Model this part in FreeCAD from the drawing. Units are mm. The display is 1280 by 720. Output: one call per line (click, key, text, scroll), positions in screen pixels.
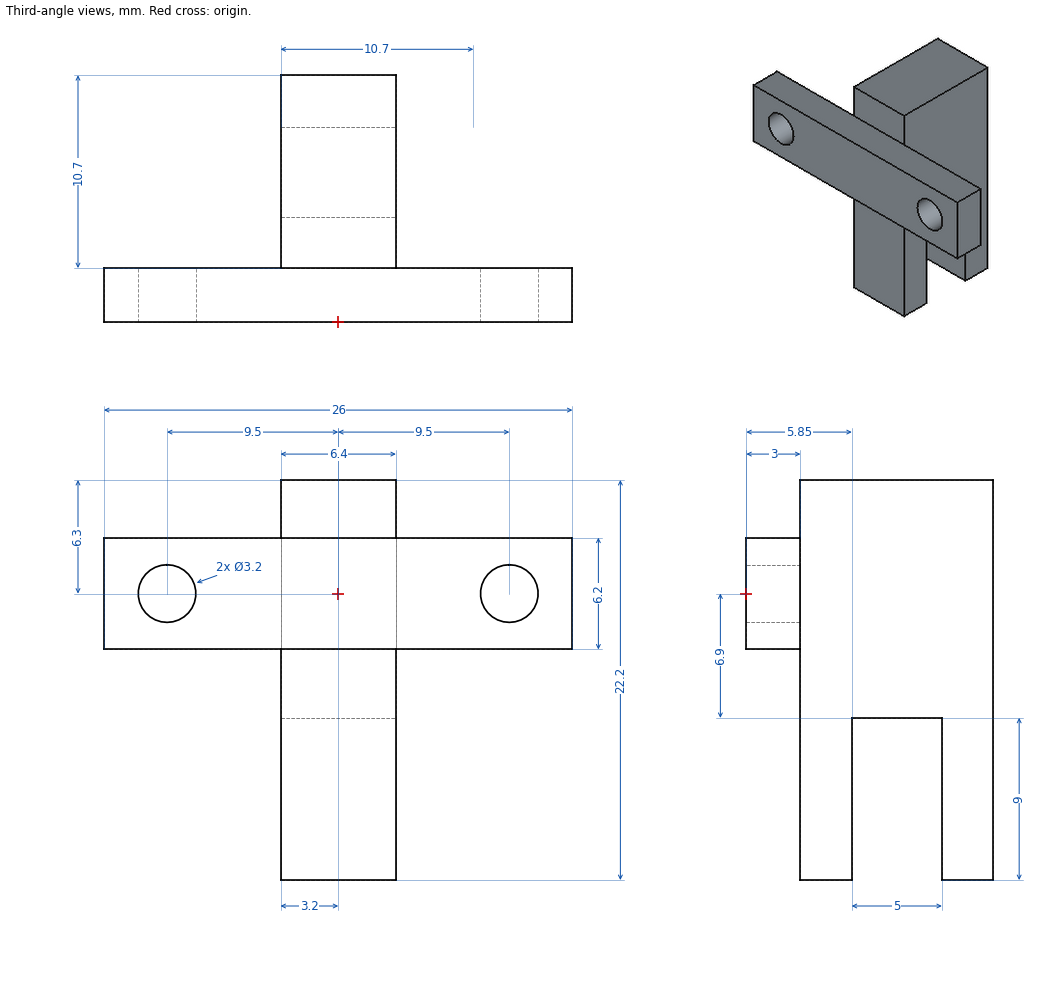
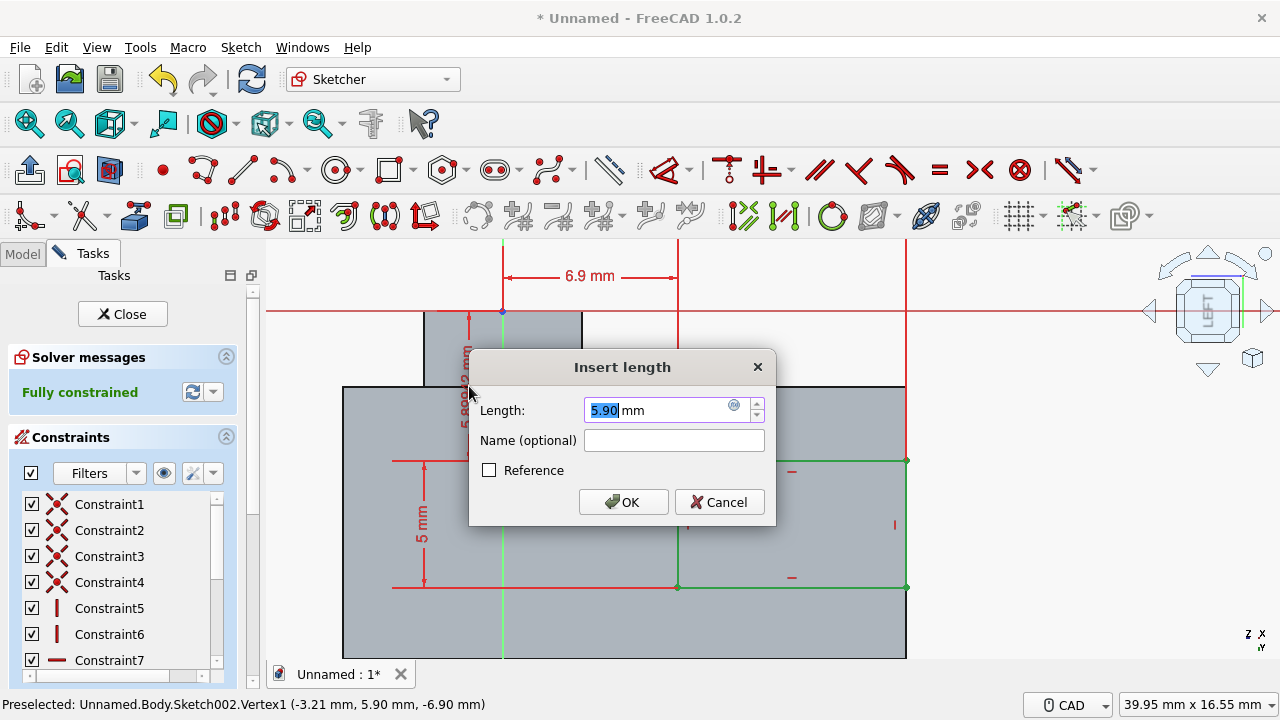
text(5.85)
key(Return)
key(Escape)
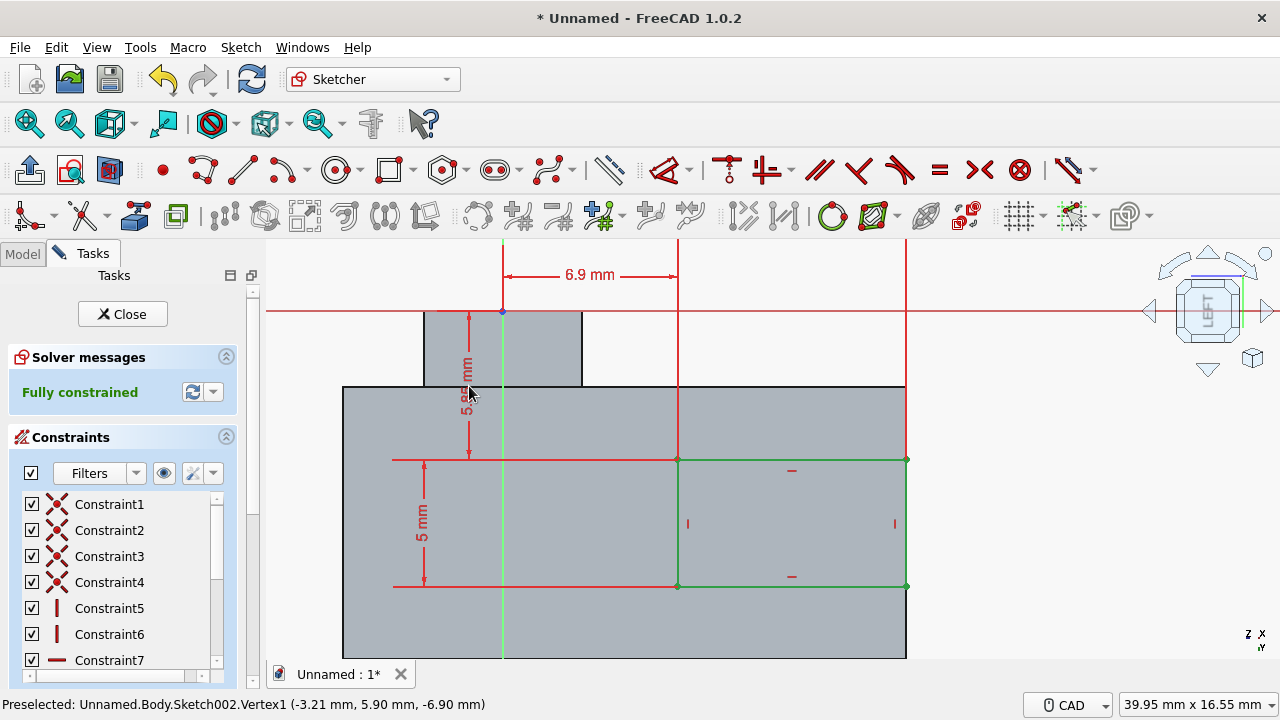
click(123, 314)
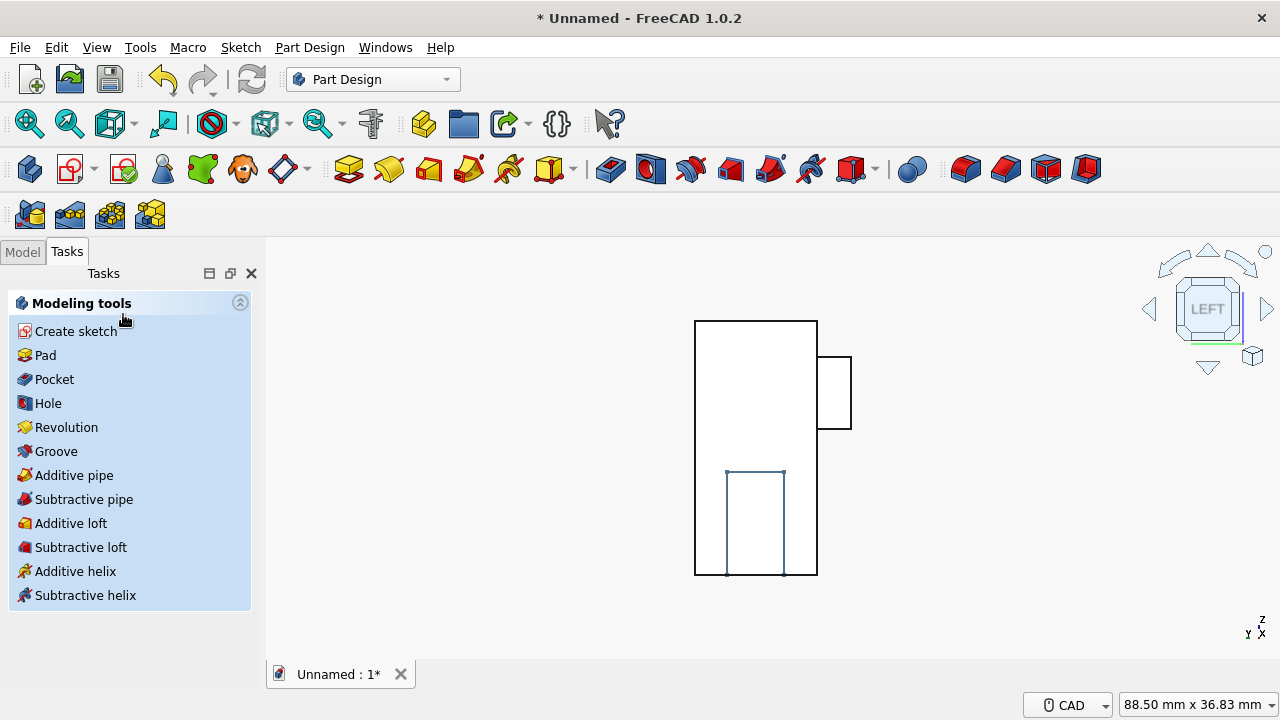
click(612, 170)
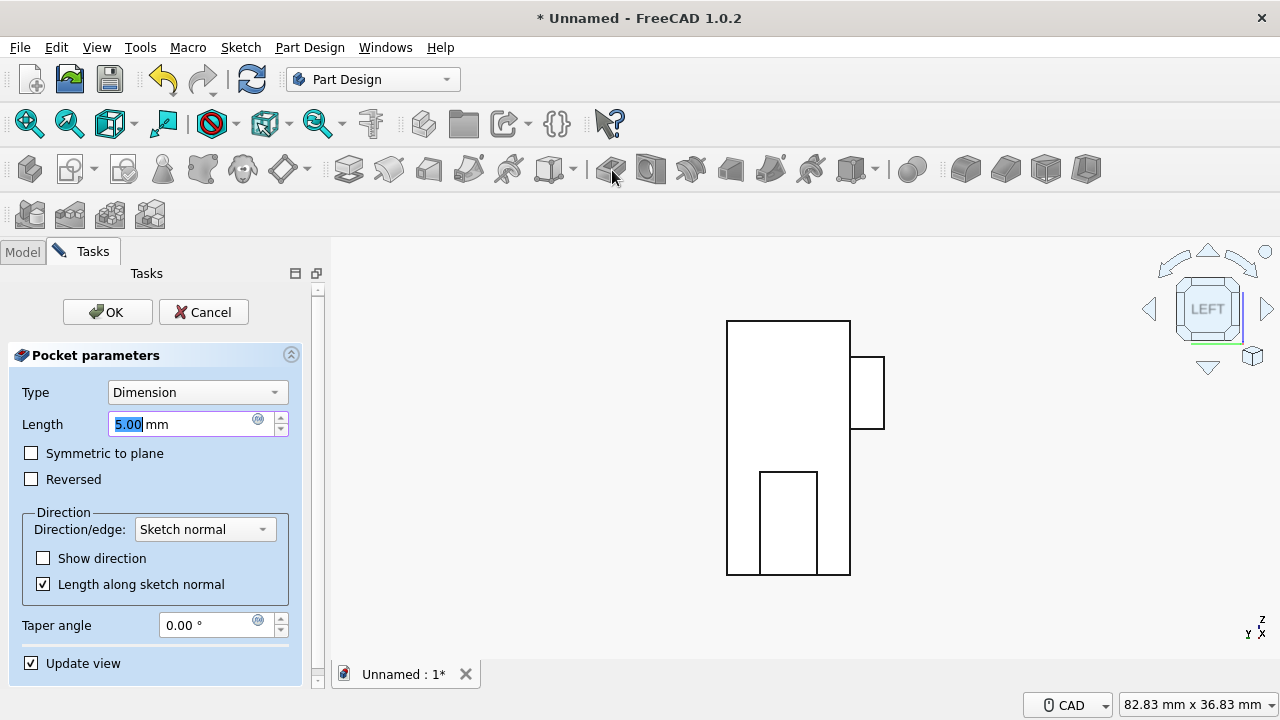
text(10.7)
key(Tab)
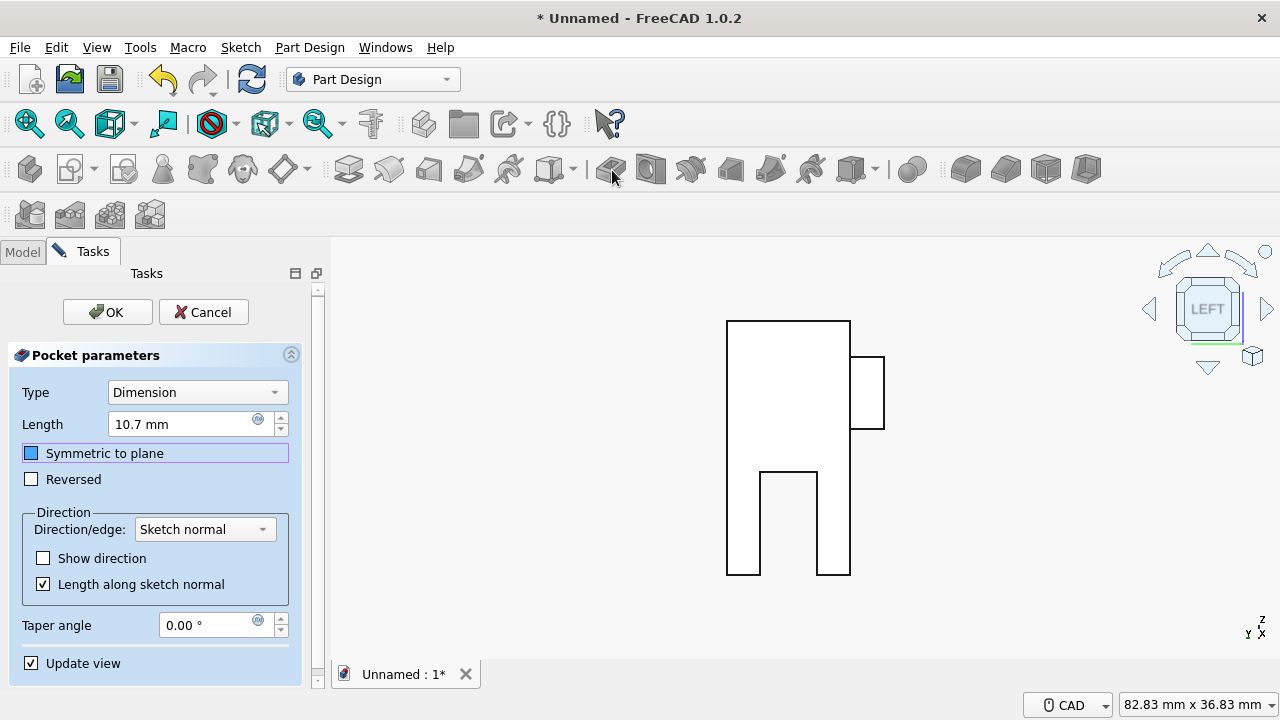
click(108, 312)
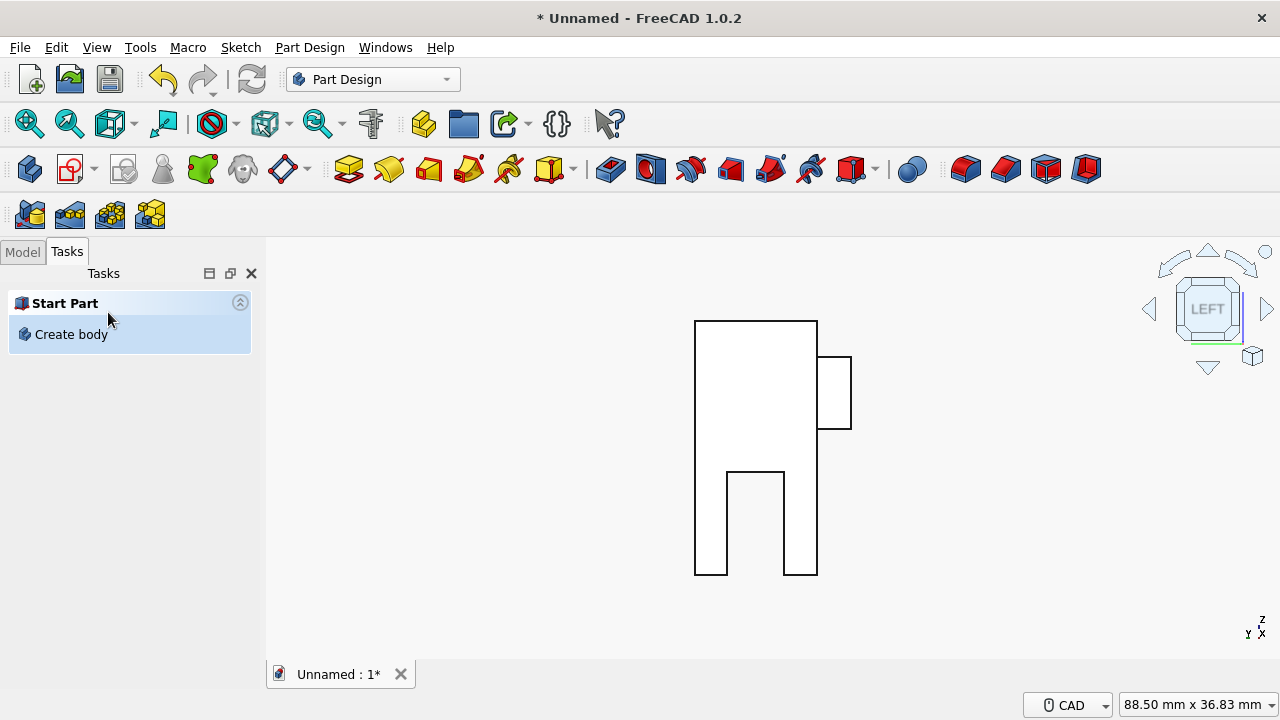
key(0)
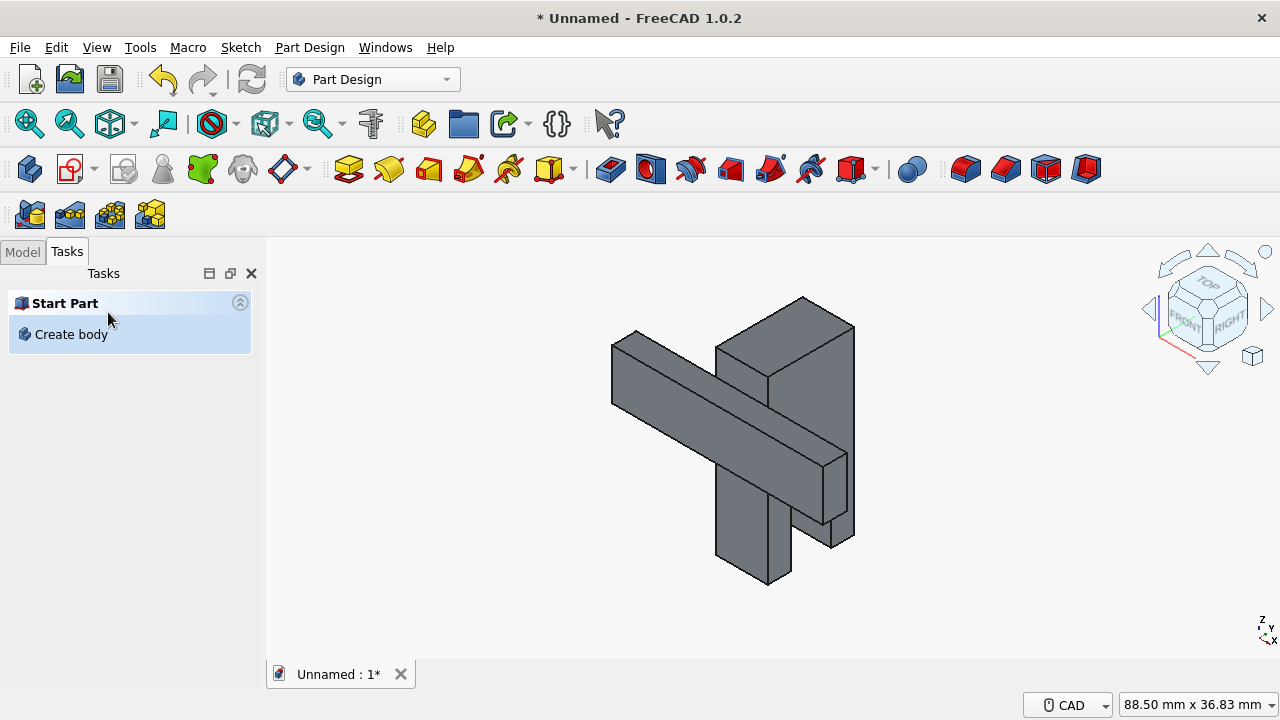
click(742, 492)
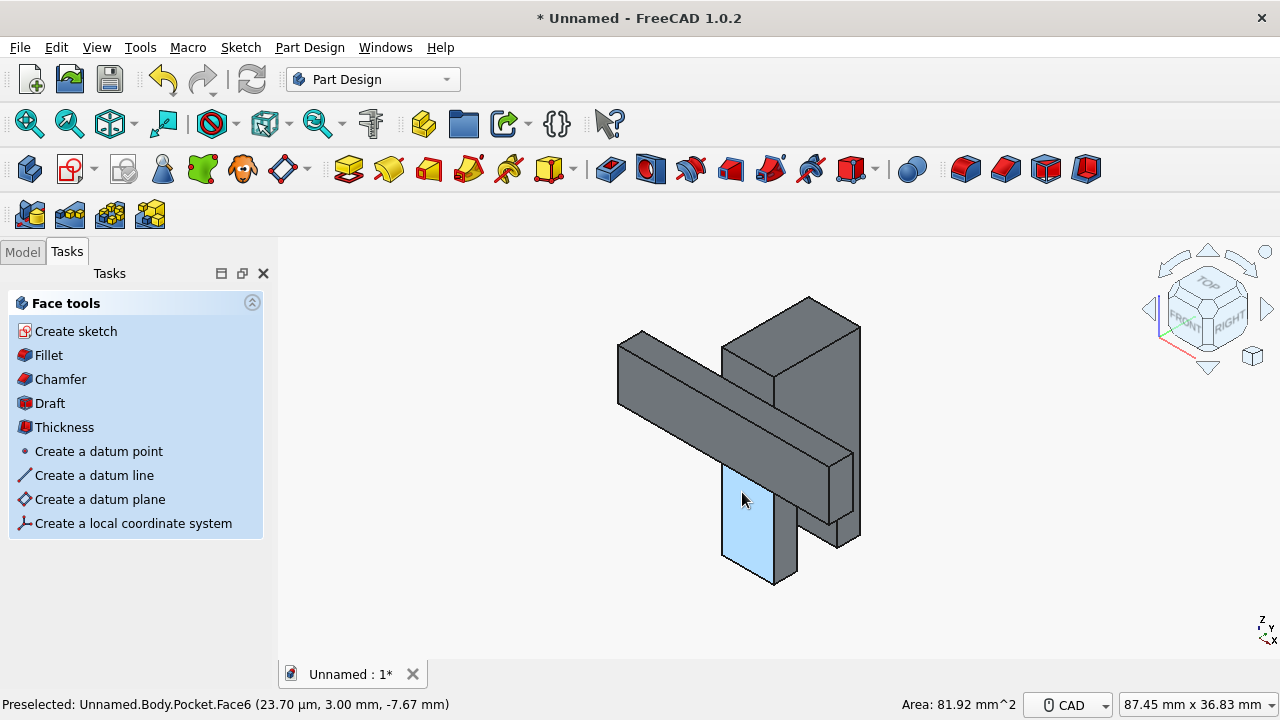
click(70, 170)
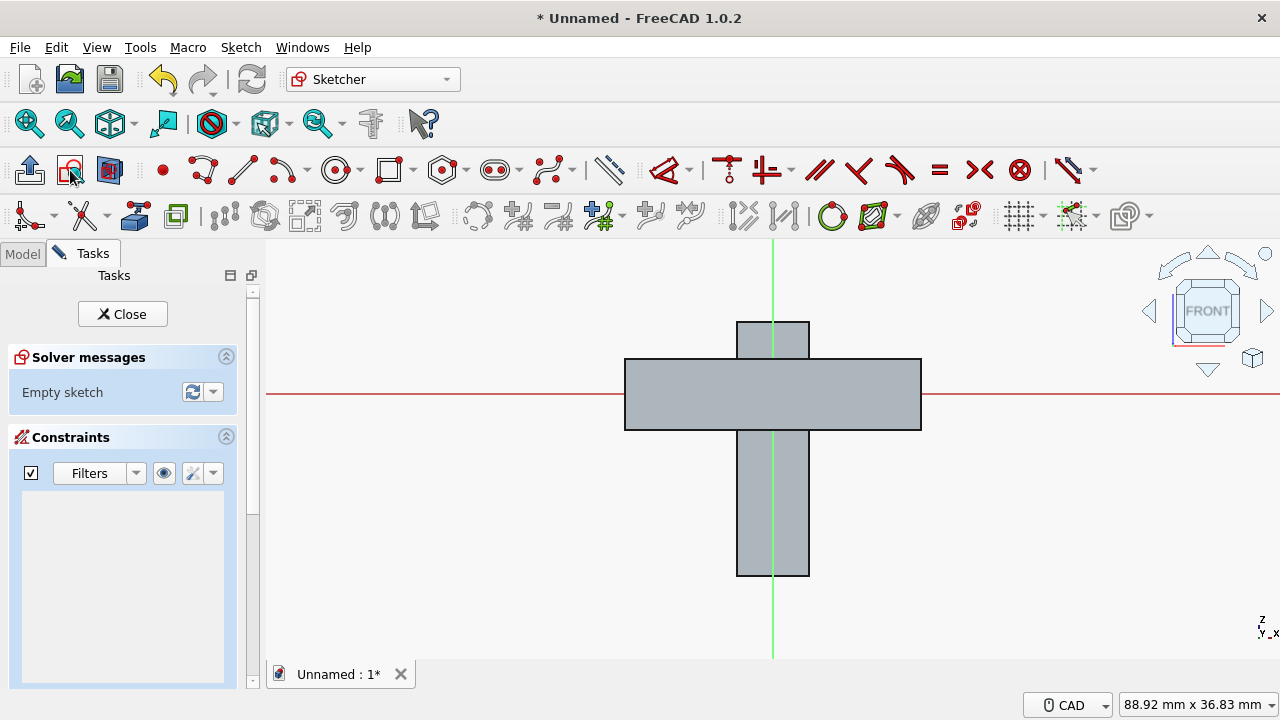
key(q)
key(s)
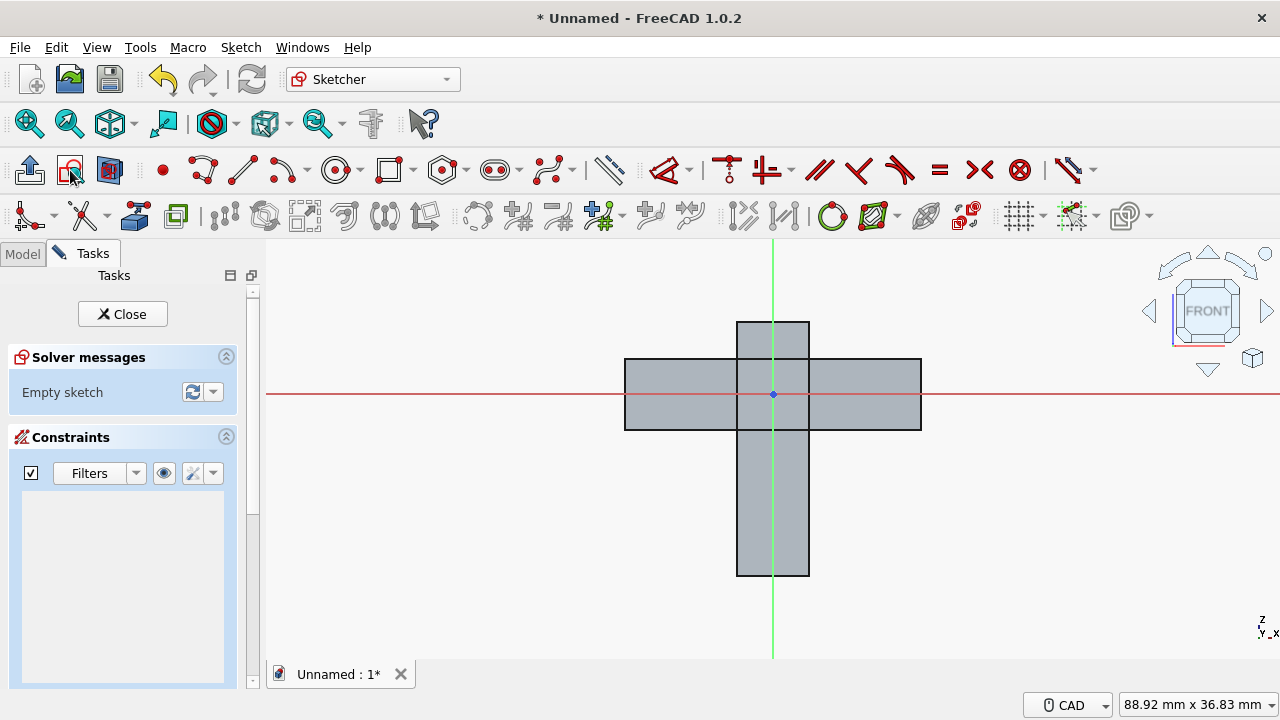
scroll(829, 350, up, 4)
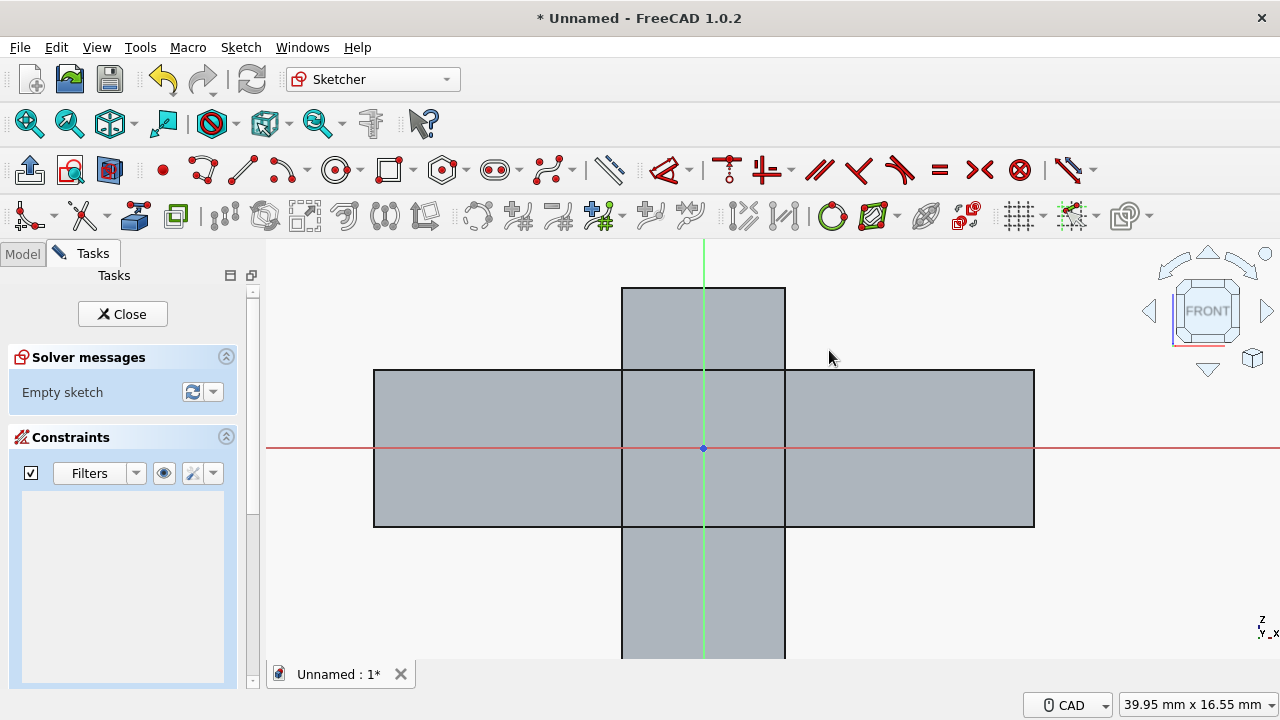
click(336, 170)